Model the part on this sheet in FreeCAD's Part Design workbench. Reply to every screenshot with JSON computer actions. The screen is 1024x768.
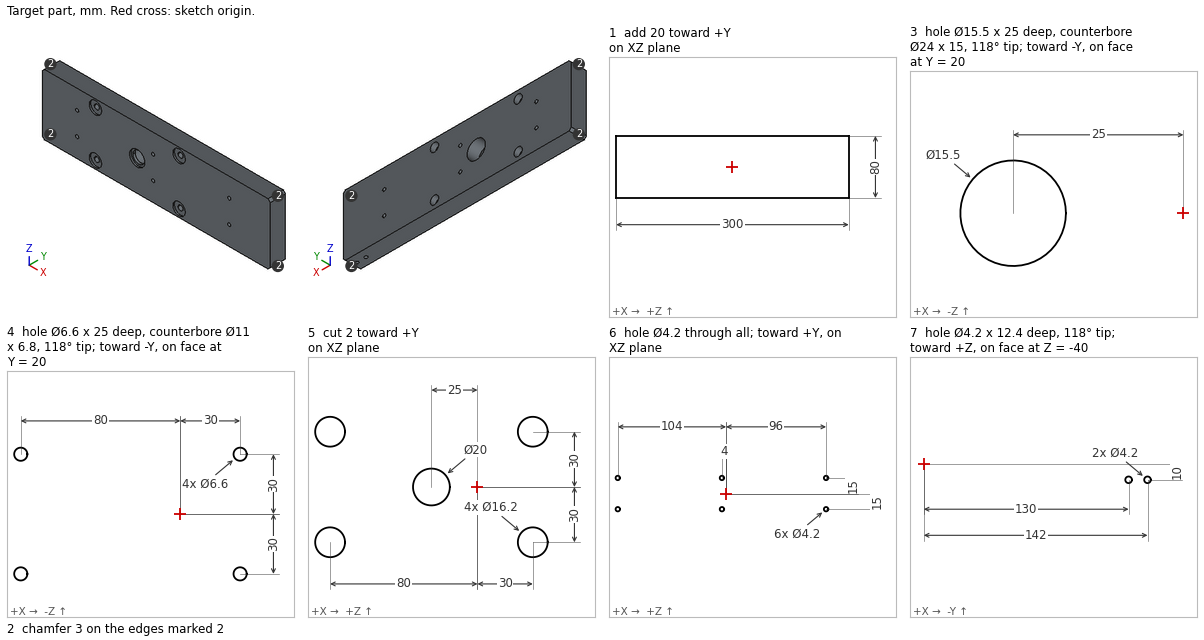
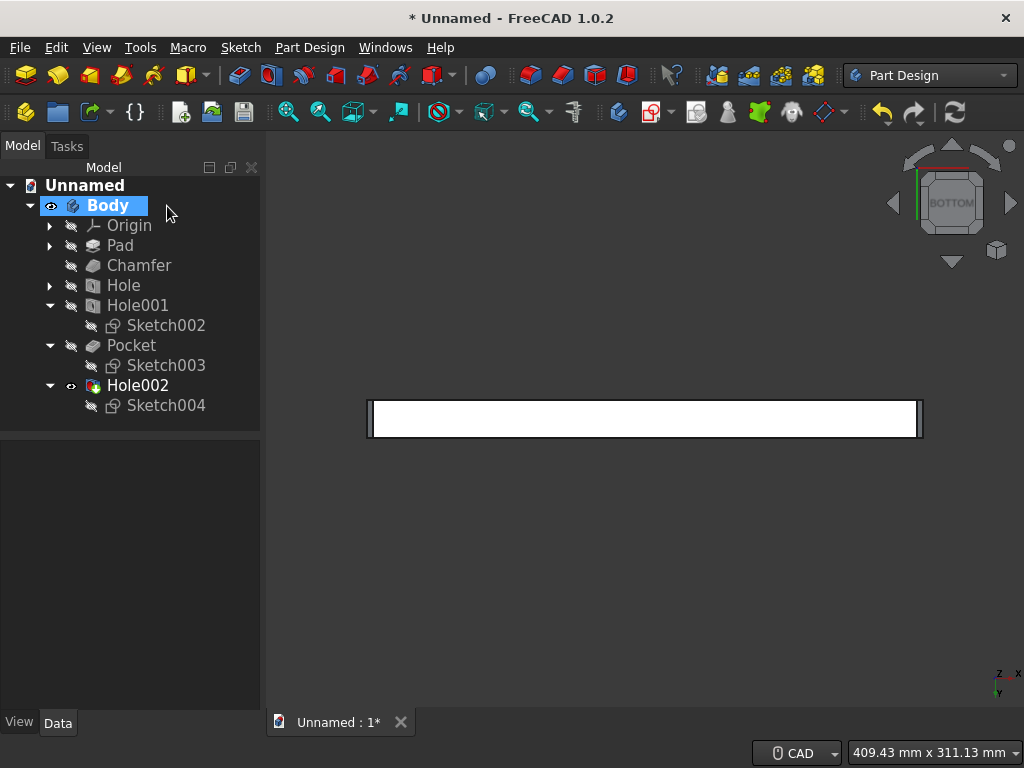
{"action": "left_click", "coordinate": [878, 418]}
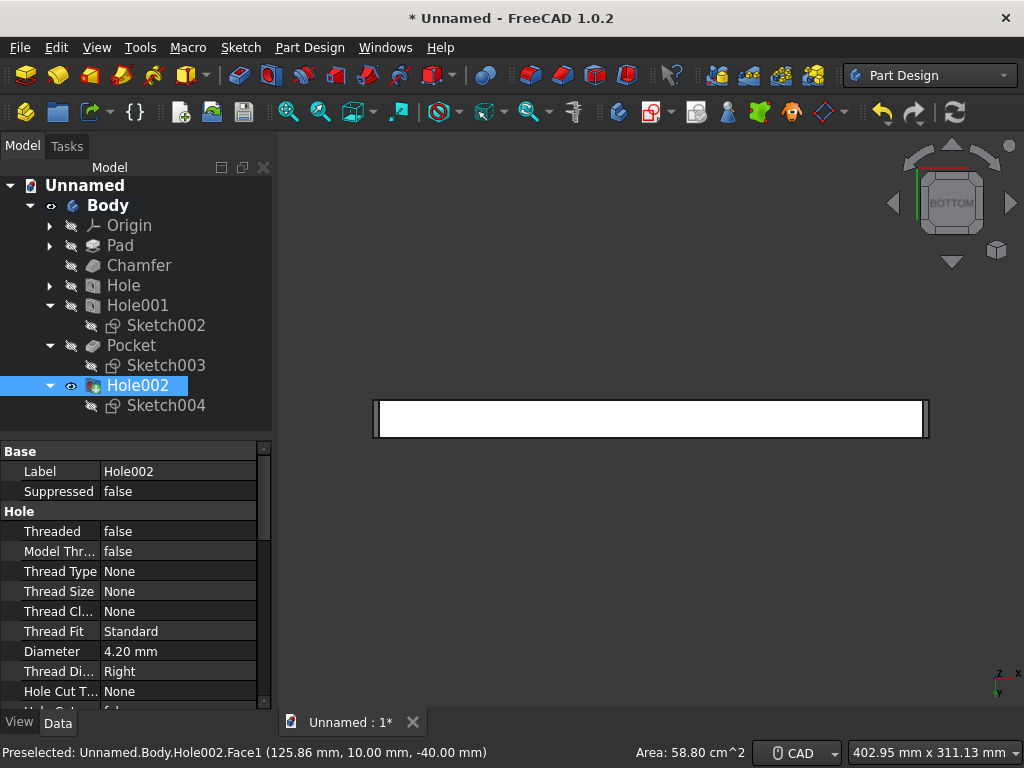
{"action": "left_click", "coordinate": [652, 112]}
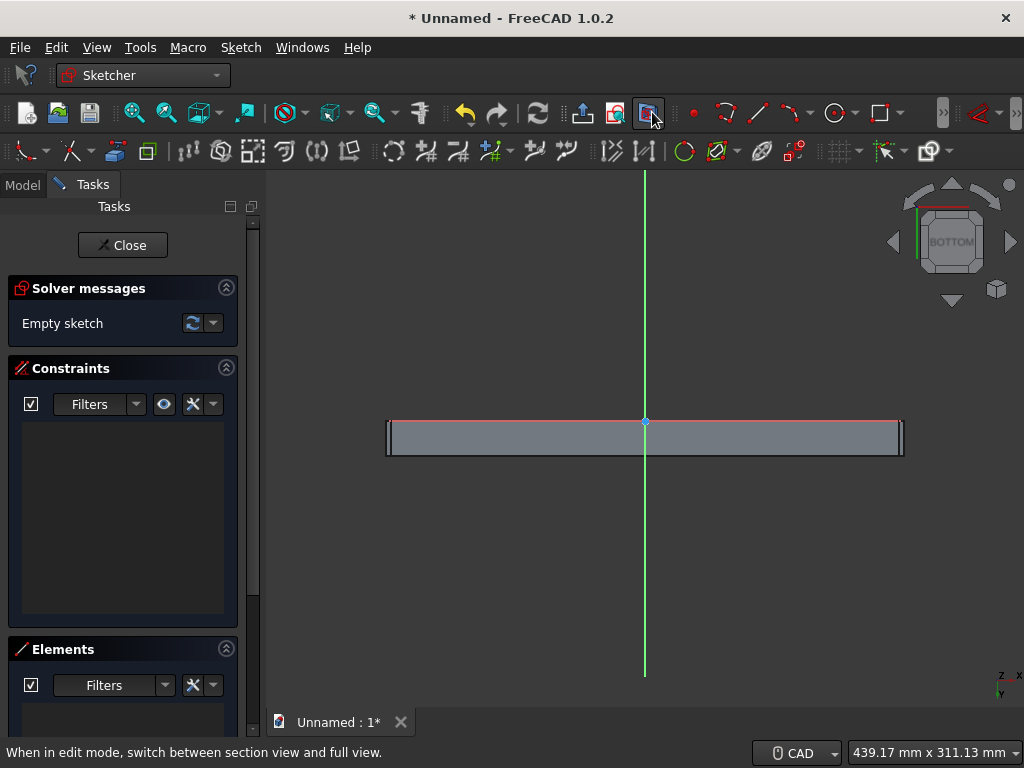
{"action": "scroll", "coordinate": [576, 438], "scroll_direction": "down", "scroll_amount": 5}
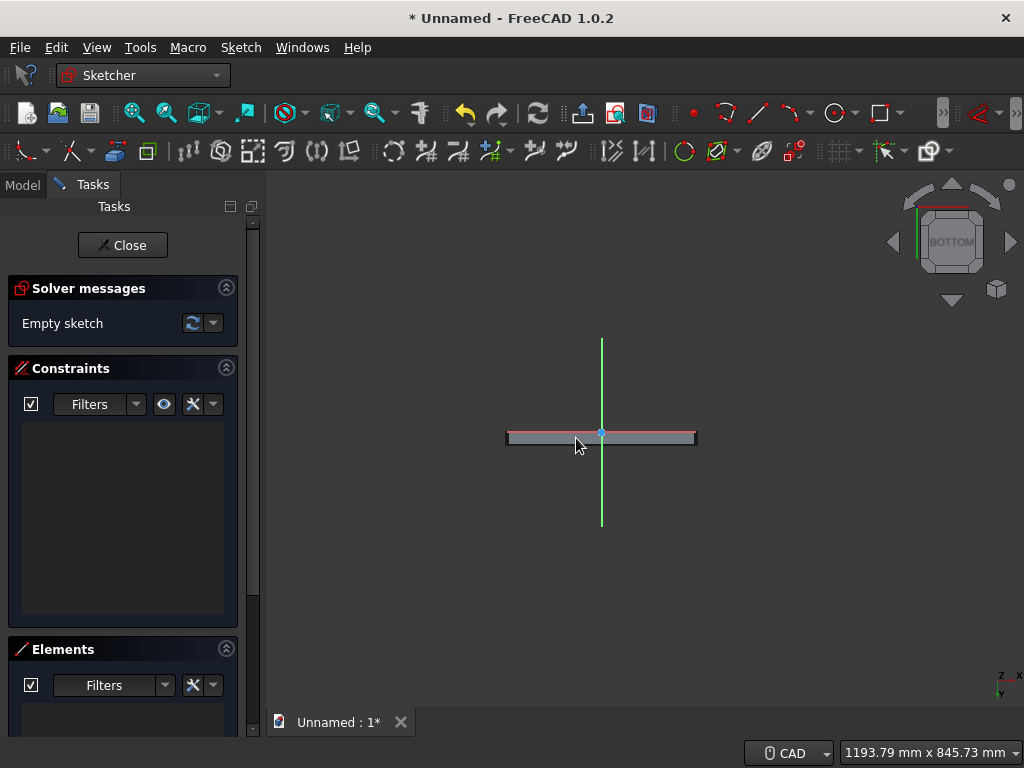
{"action": "scroll", "coordinate": [694, 439], "scroll_direction": "up", "scroll_amount": 15}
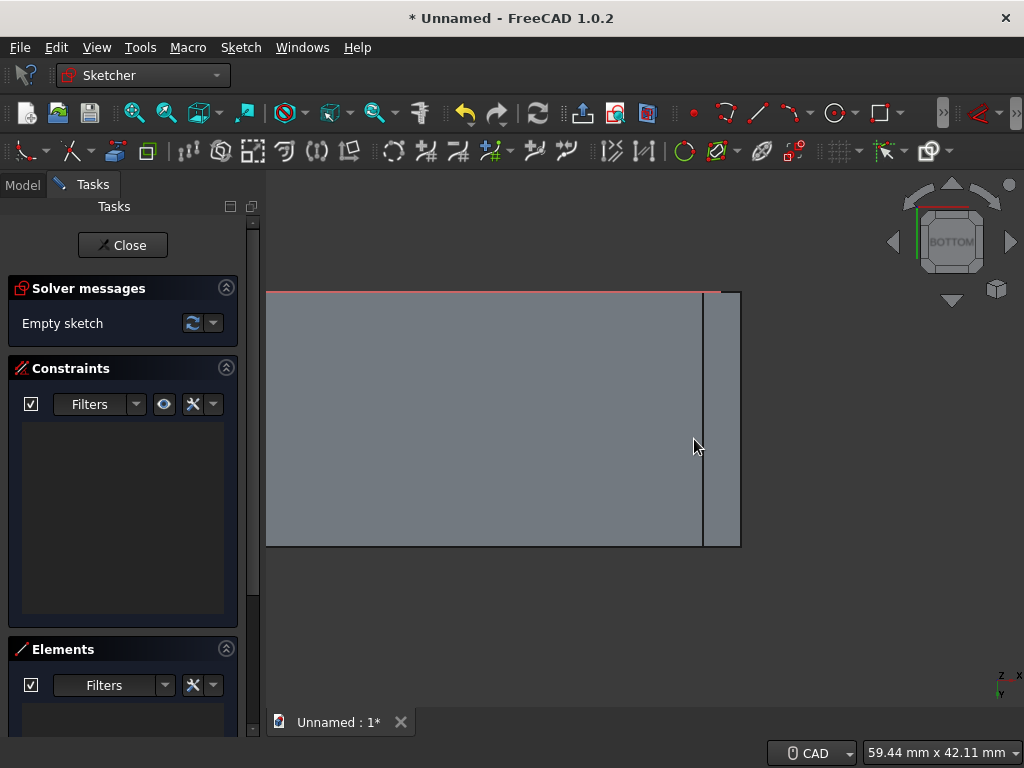
{"action": "scroll", "coordinate": [546, 396], "scroll_direction": "up", "scroll_amount": 3}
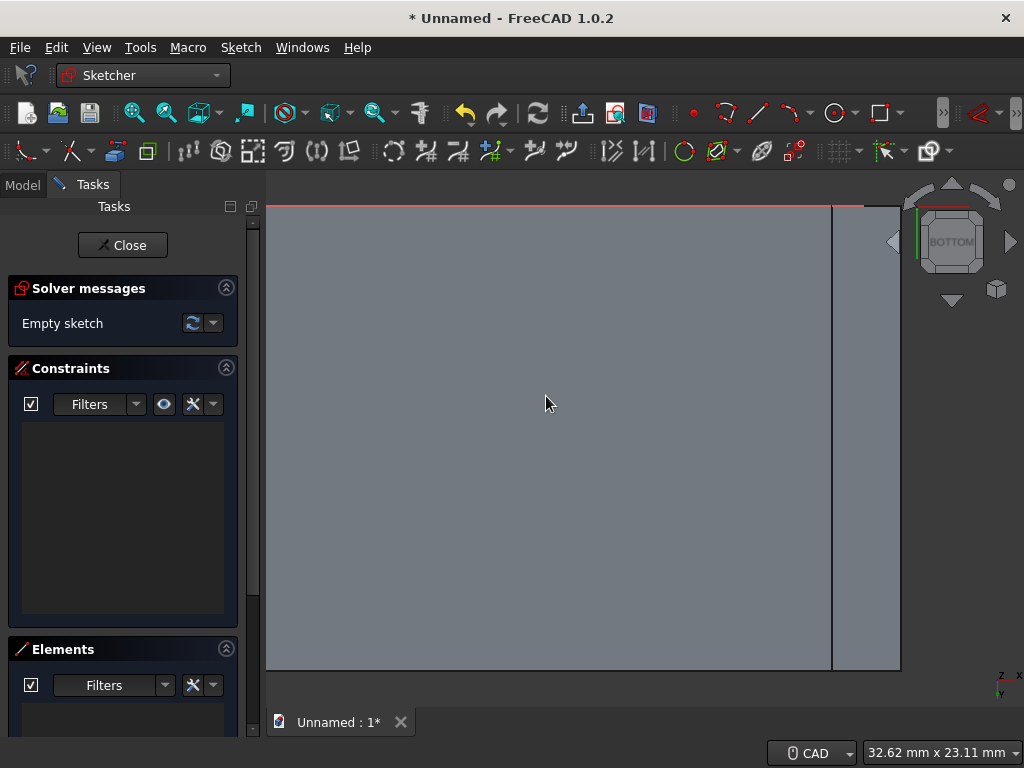
{"action": "left_click", "coordinate": [836, 114]}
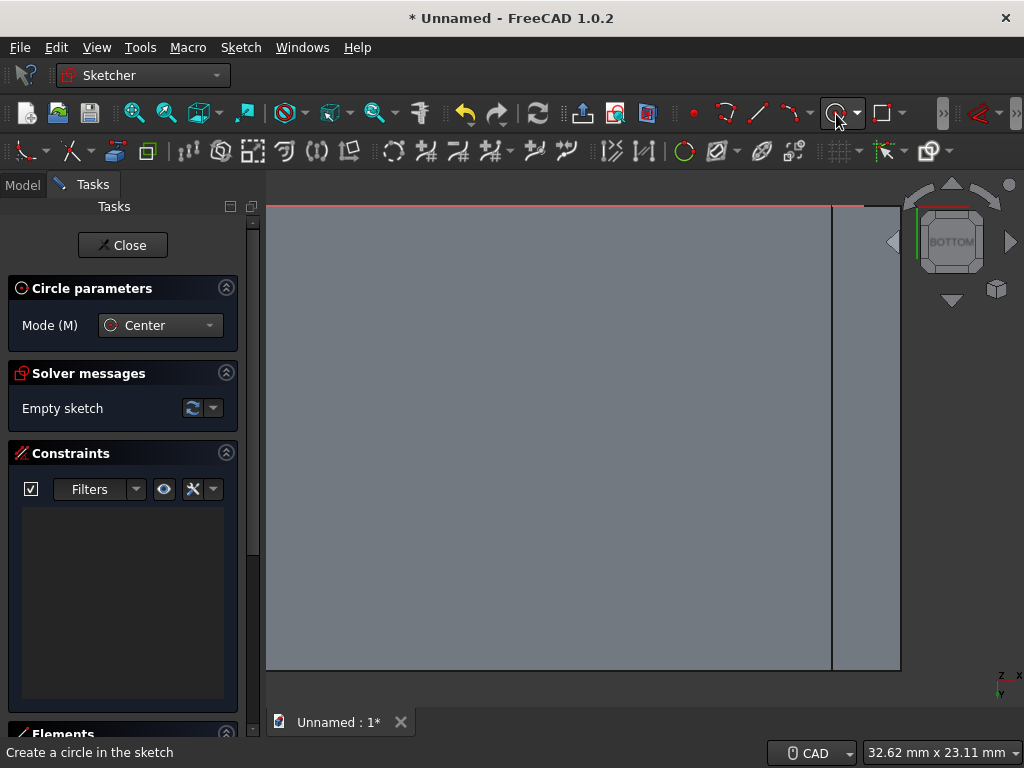
{"action": "left_click", "coordinate": [715, 438]}
{"action": "mouse_move", "coordinate": [750, 404]}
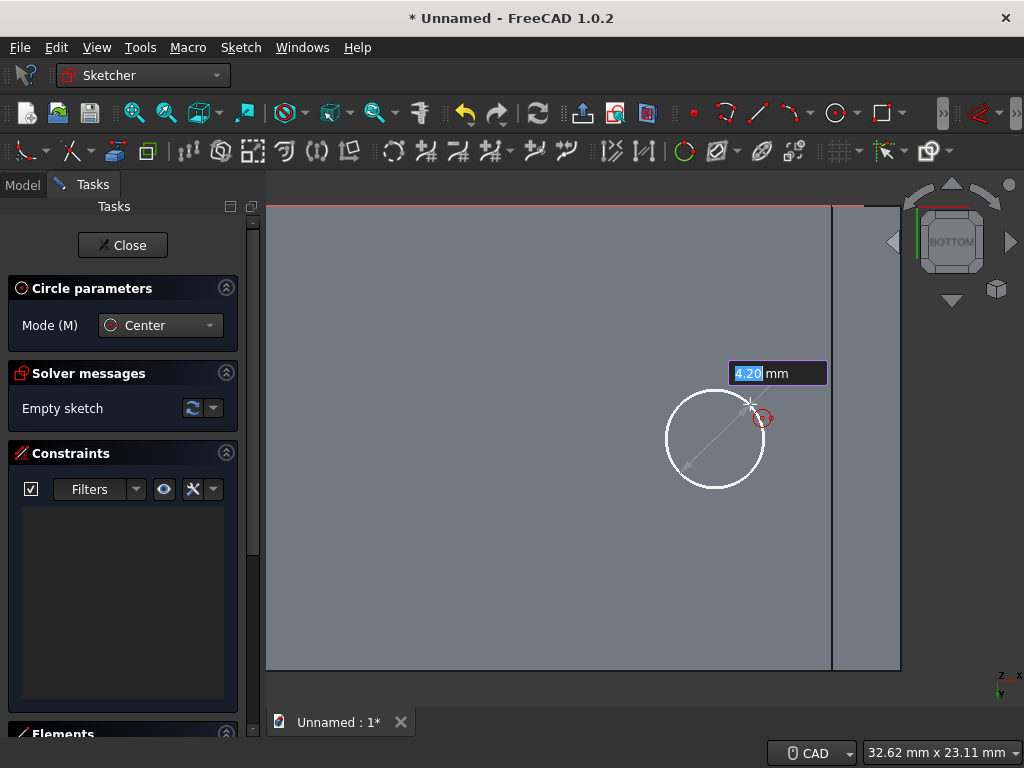
{"action": "type", "text": "4.2"}
{"action": "key", "text": "Return"}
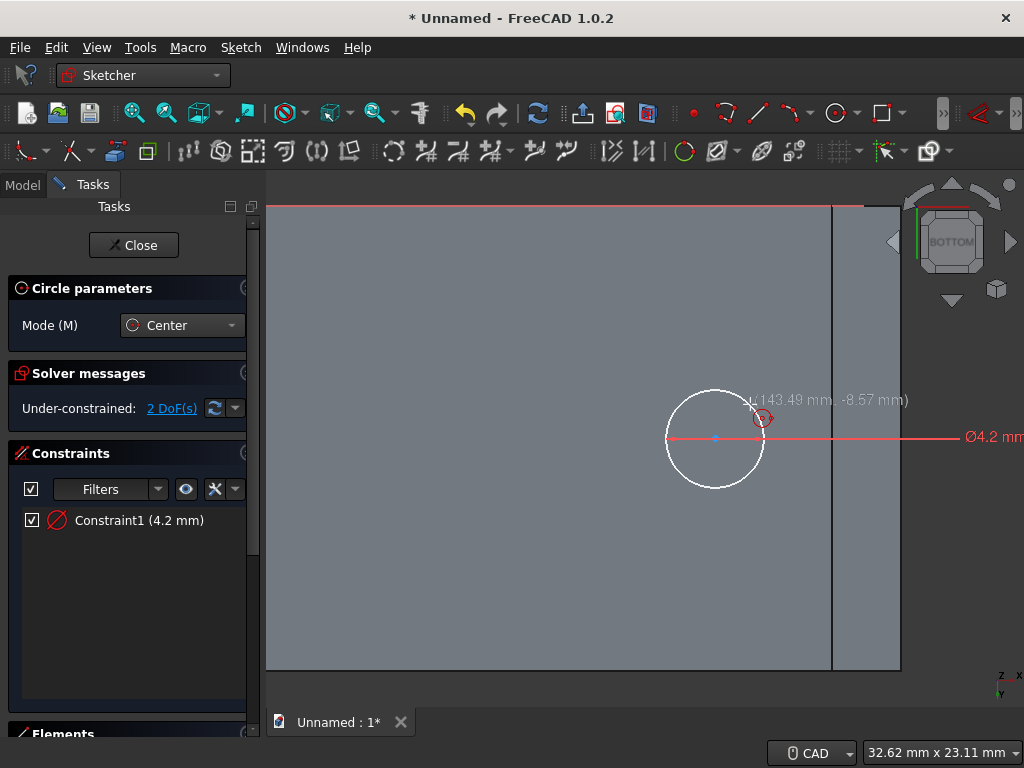
{"action": "left_click", "coordinate": [437, 438]}
{"action": "mouse_move", "coordinate": [471, 404]}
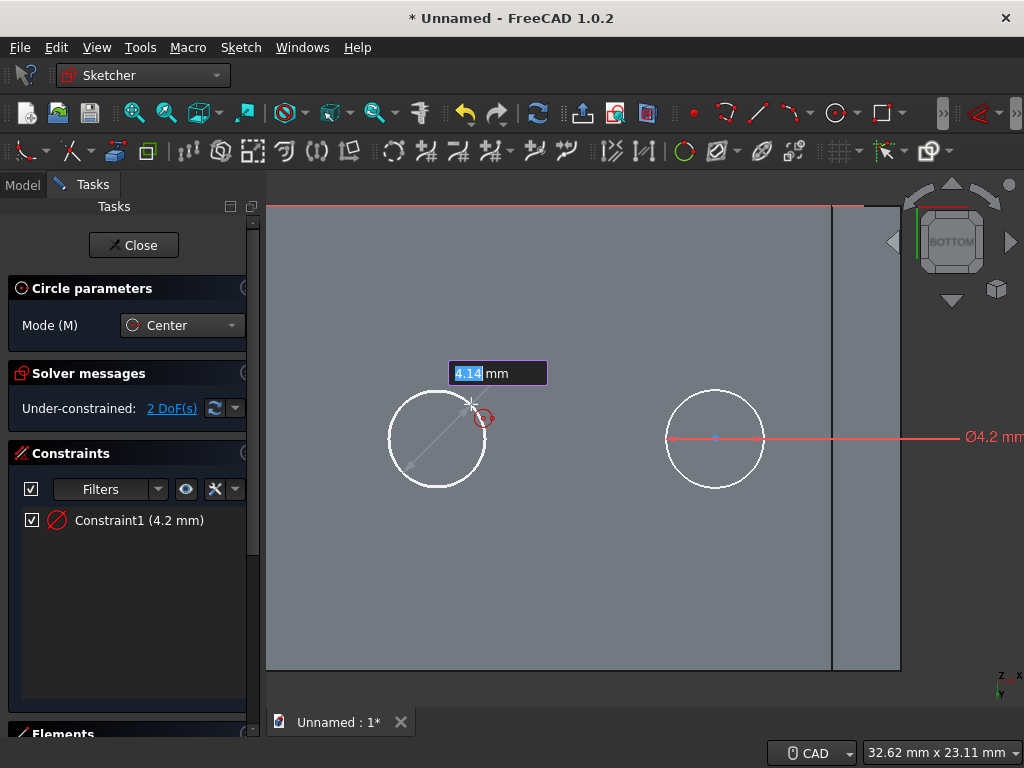
{"action": "type", "text": "4.2"}
{"action": "key", "text": "Return"}
{"action": "key", "text": "Escape"}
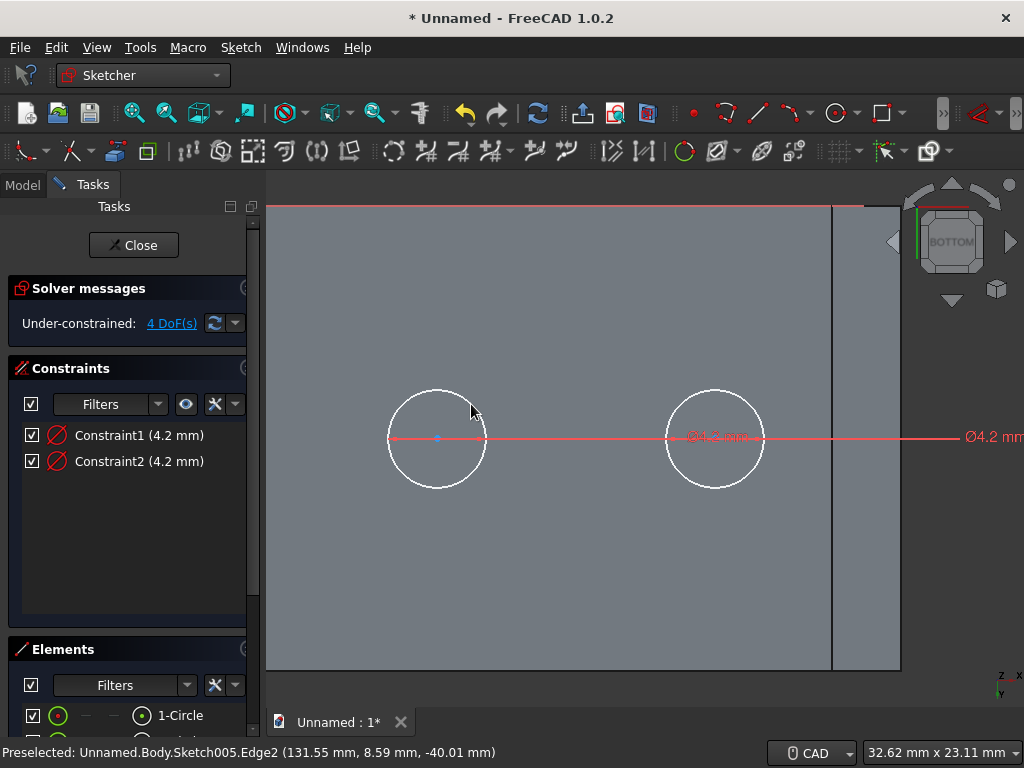
{"action": "left_click", "coordinate": [715, 439]}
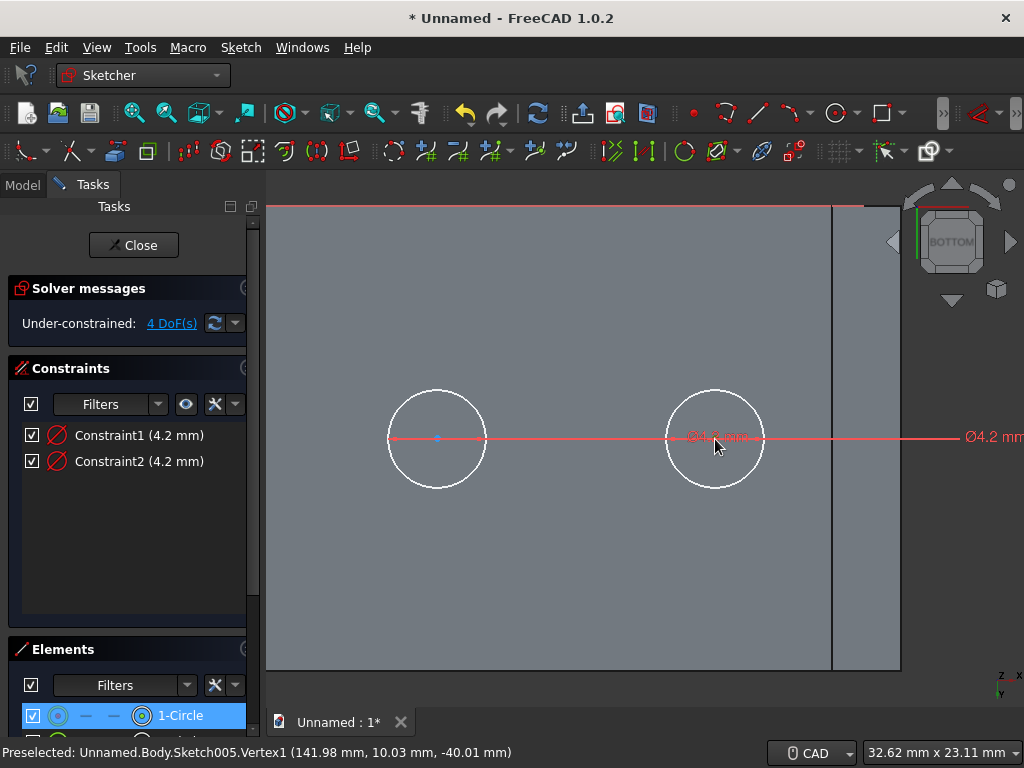
{"action": "left_click", "coordinate": [437, 439]}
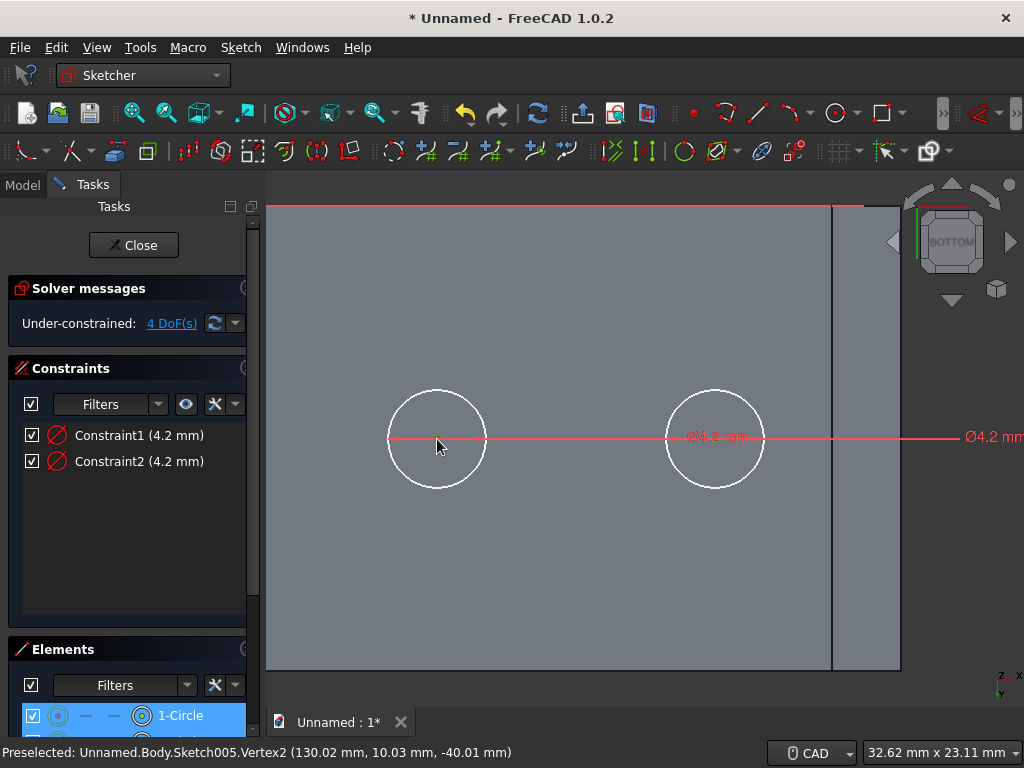
{"action": "key", "text": "h"}